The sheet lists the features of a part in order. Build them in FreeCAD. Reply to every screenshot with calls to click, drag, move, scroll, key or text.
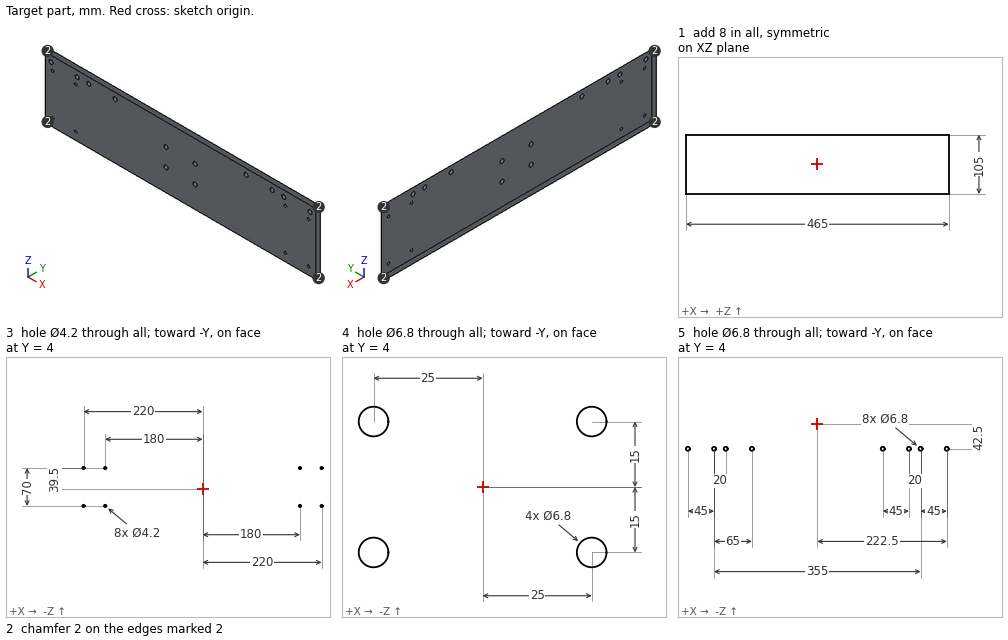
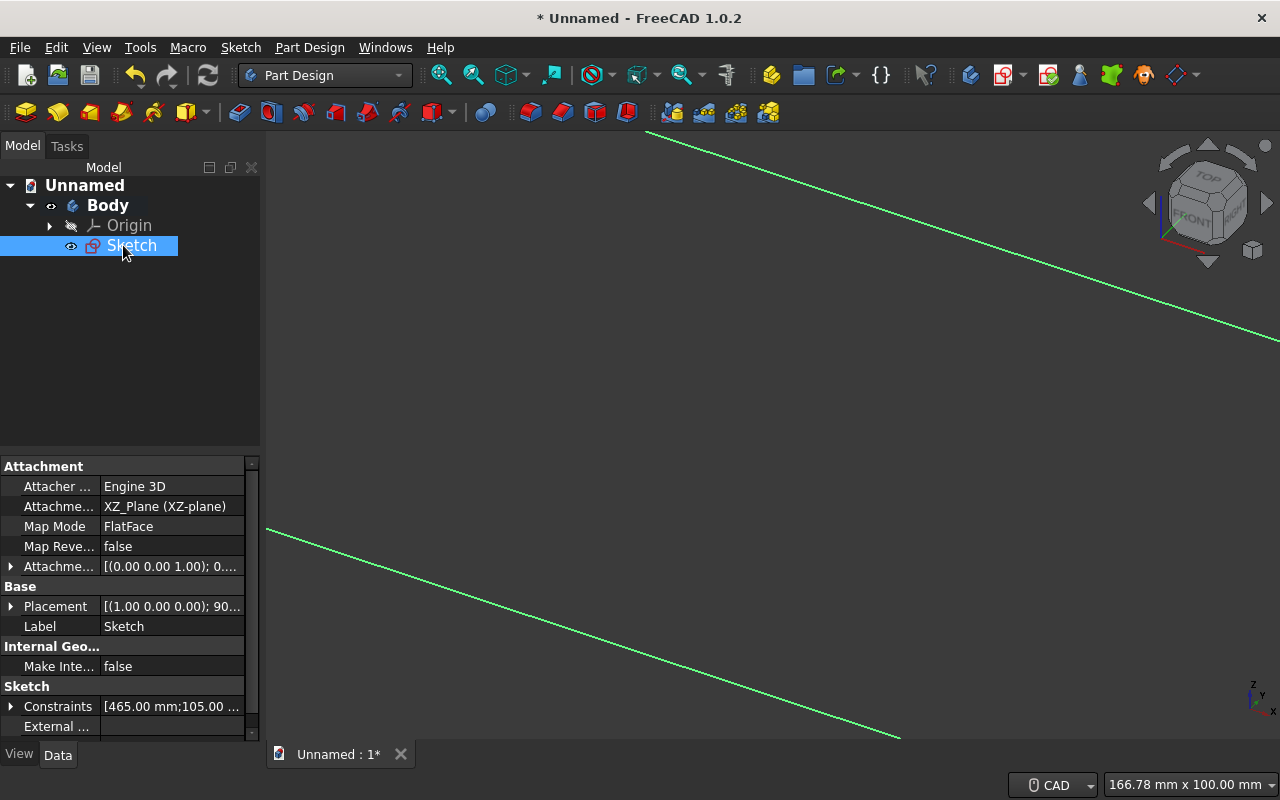
click(26, 112)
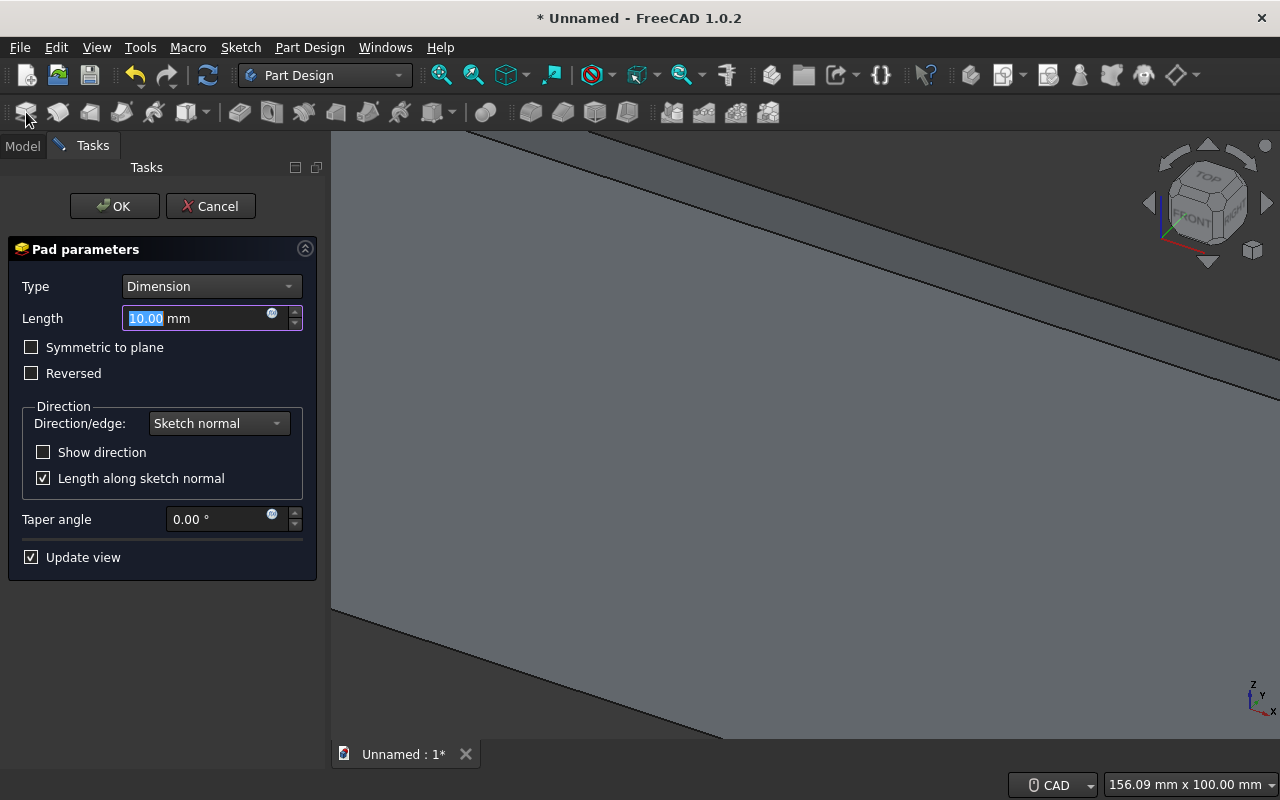
text(8)
key(Tab)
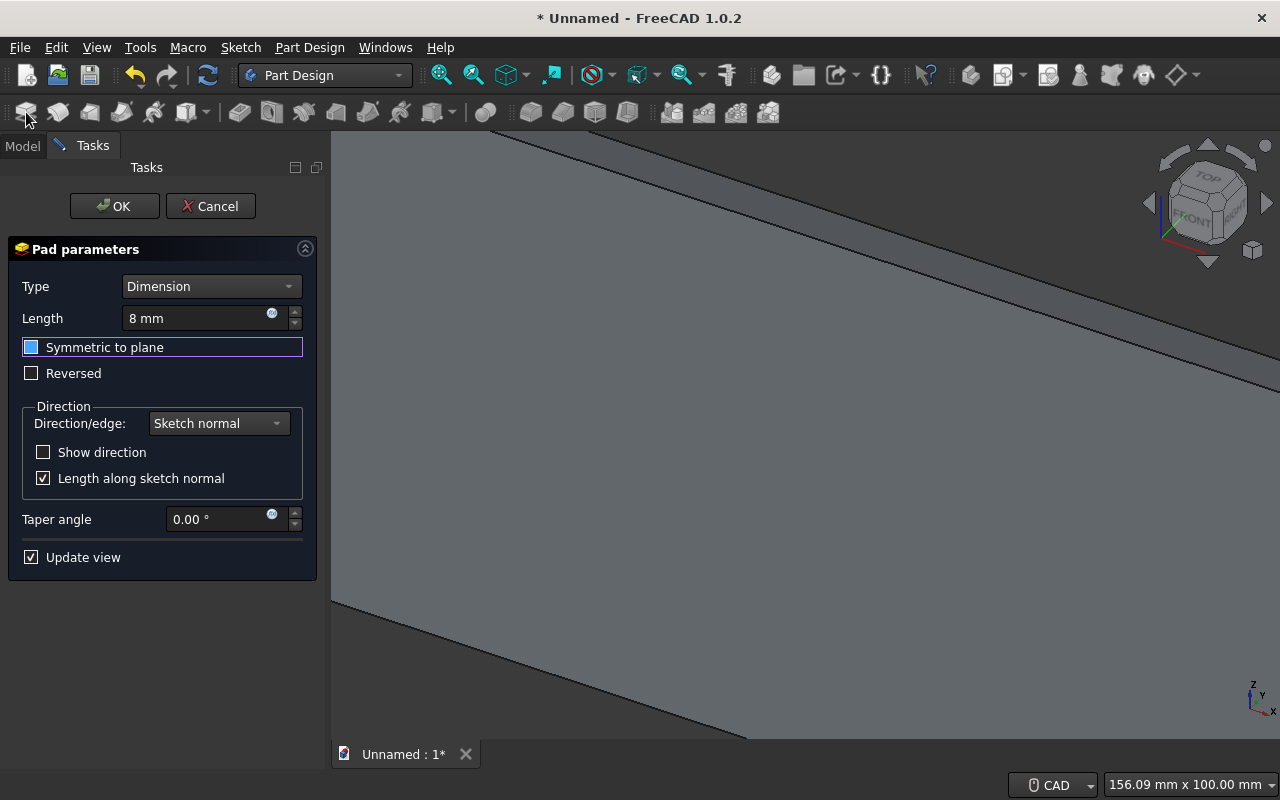
click(30, 347)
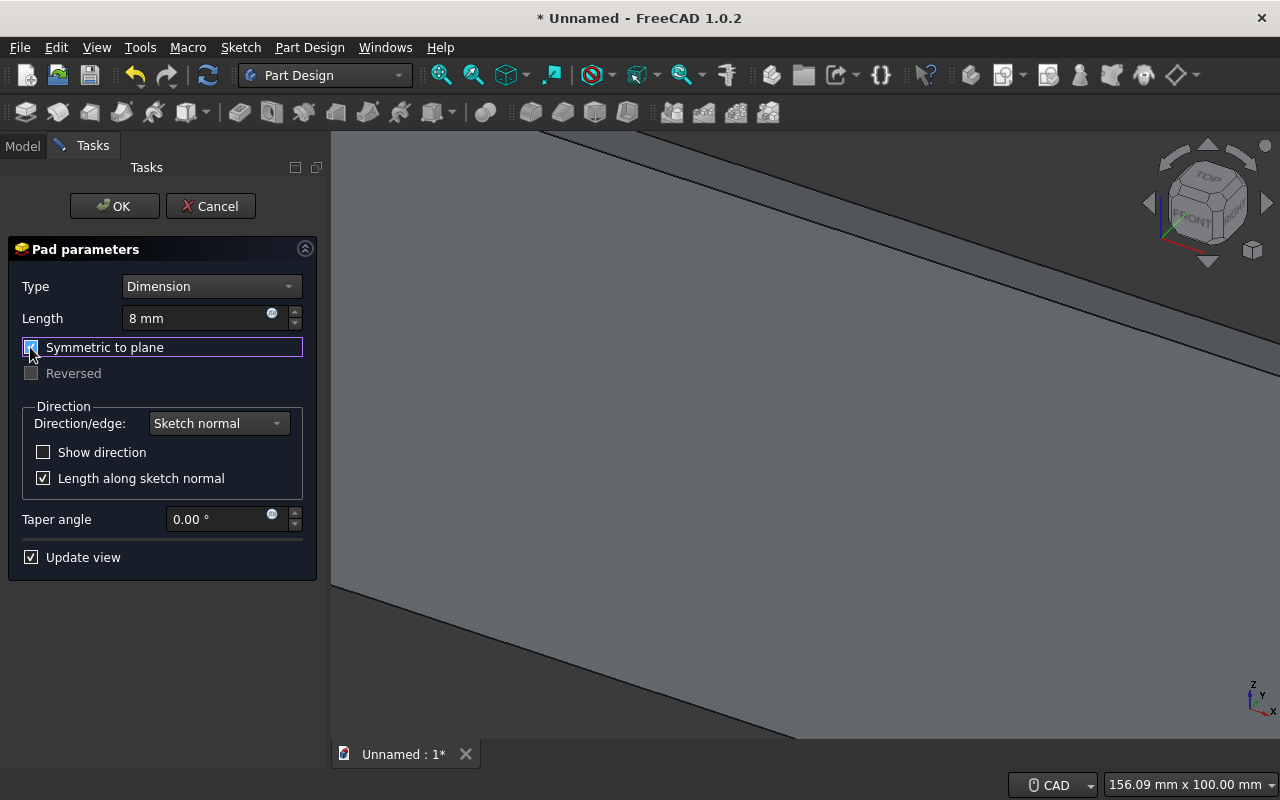
click(115, 206)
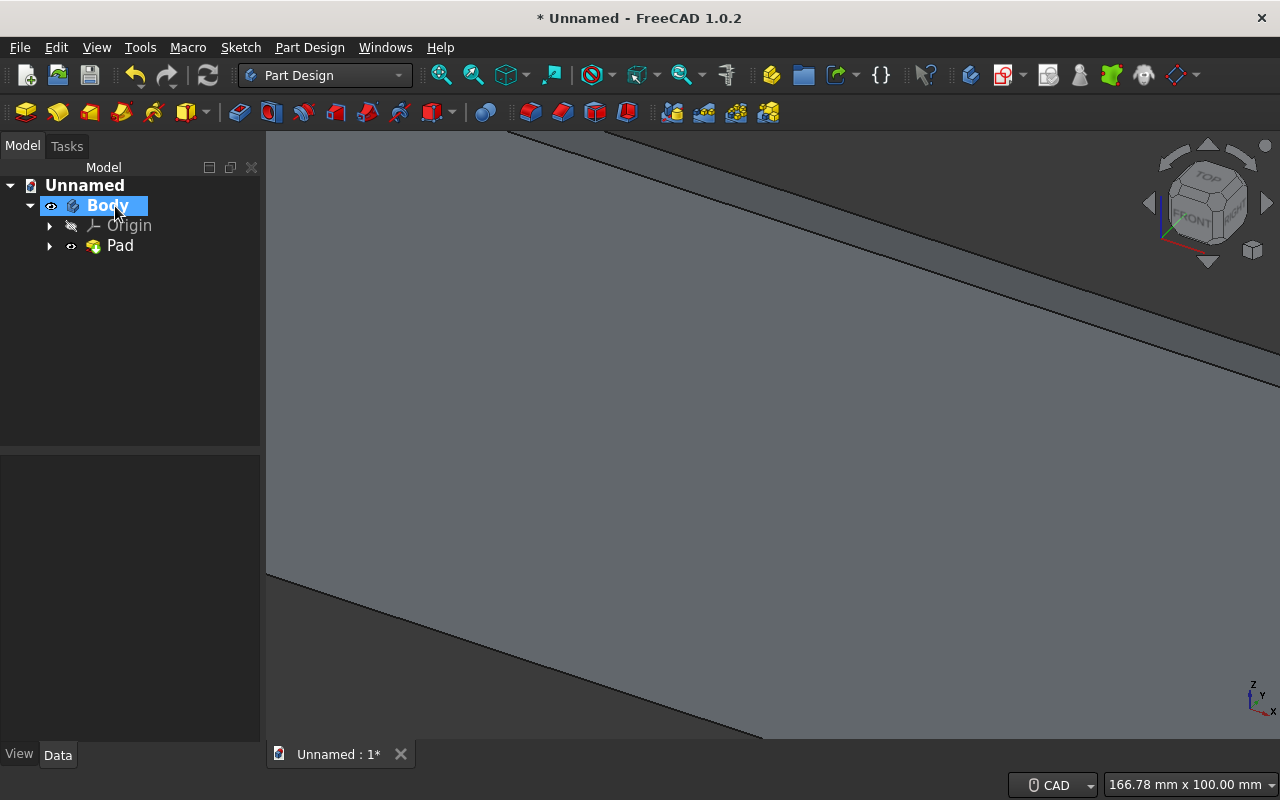
click(442, 76)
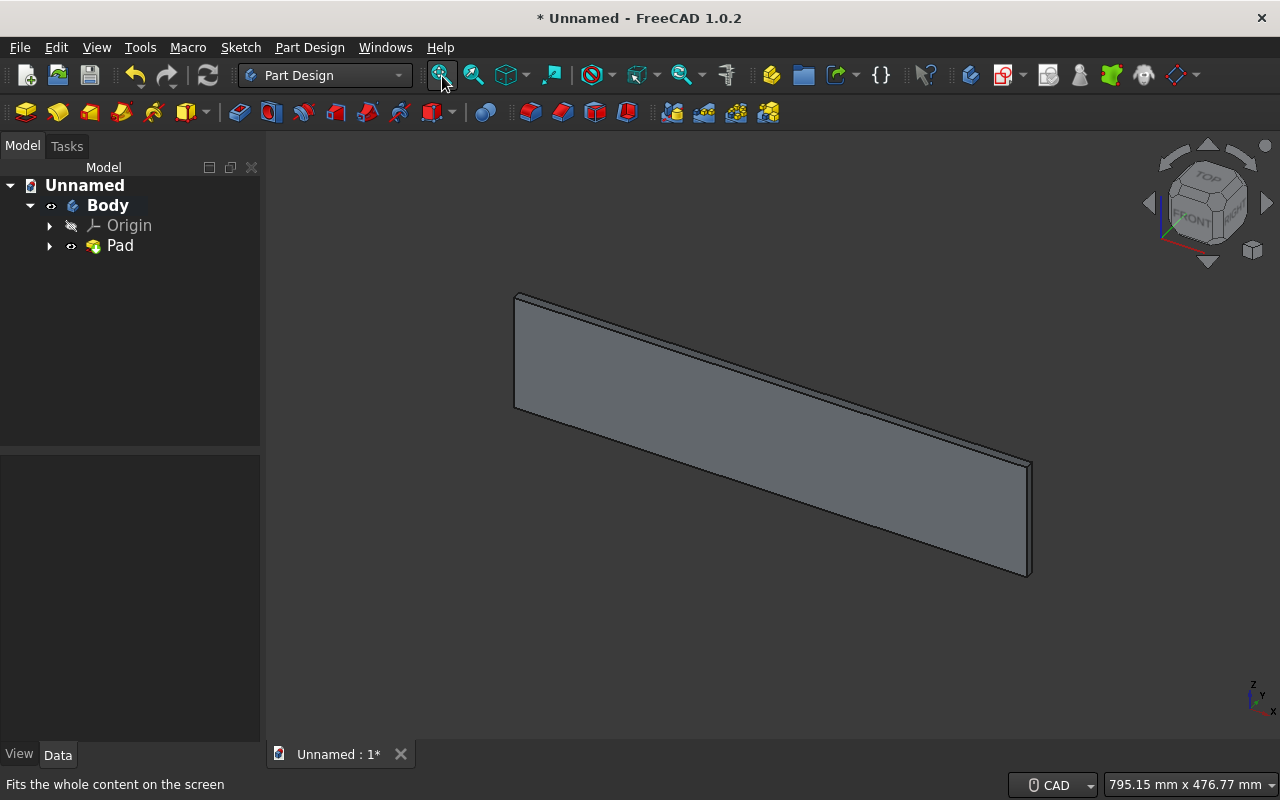
scroll(1030, 464, up, 7)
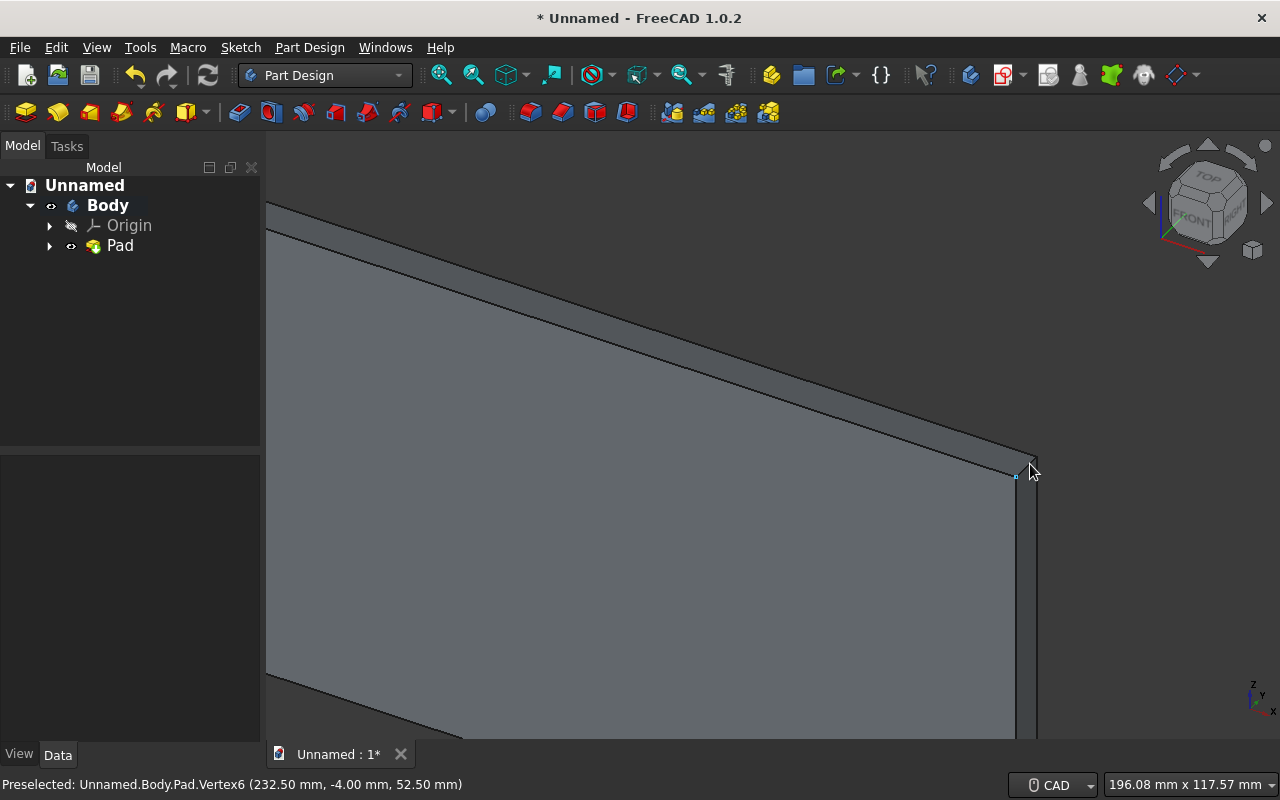
click(1027, 466)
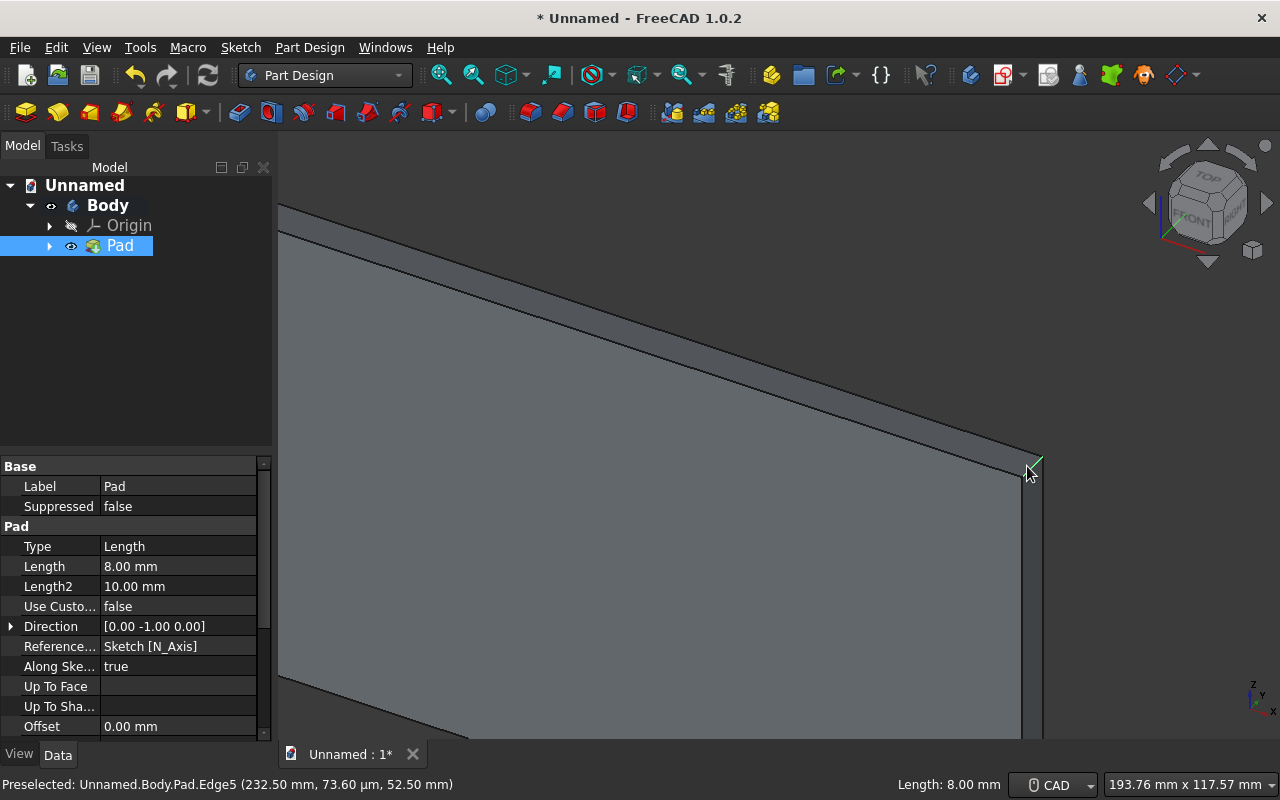
click(442, 76)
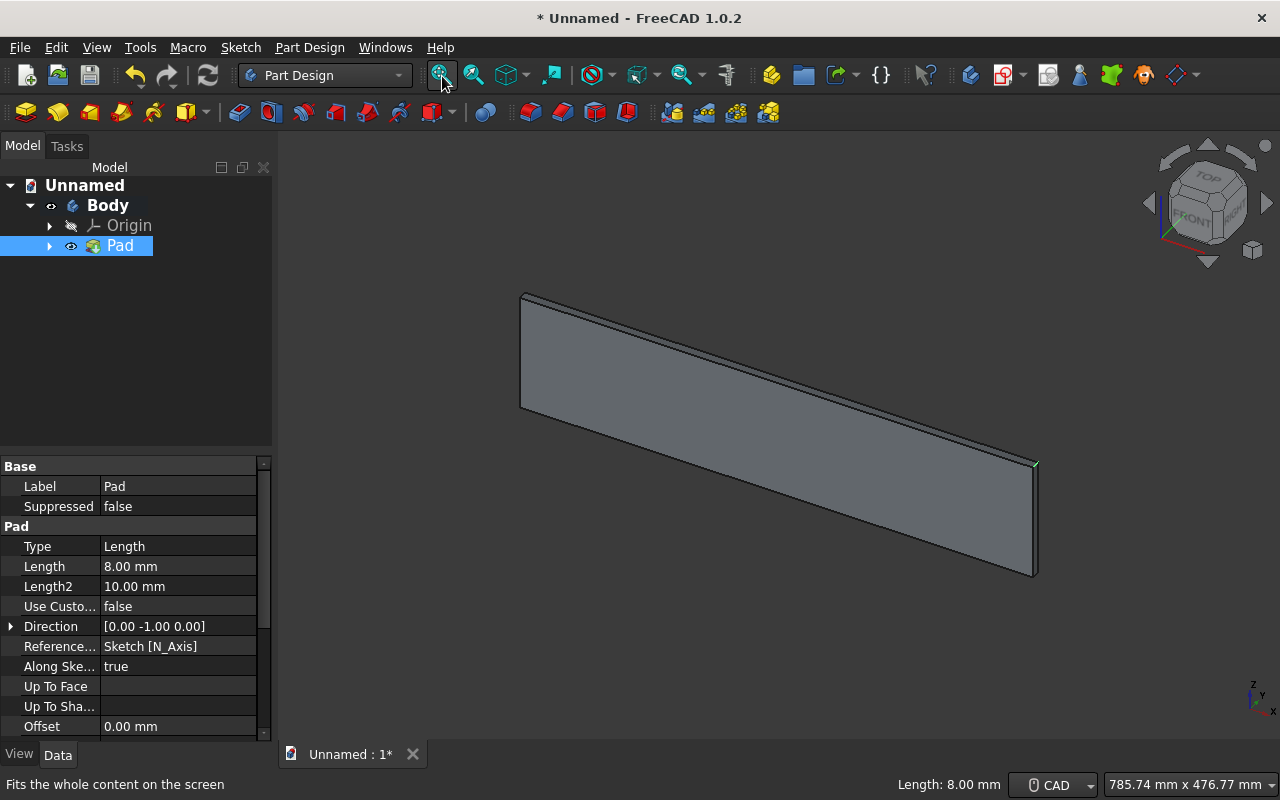
key(0)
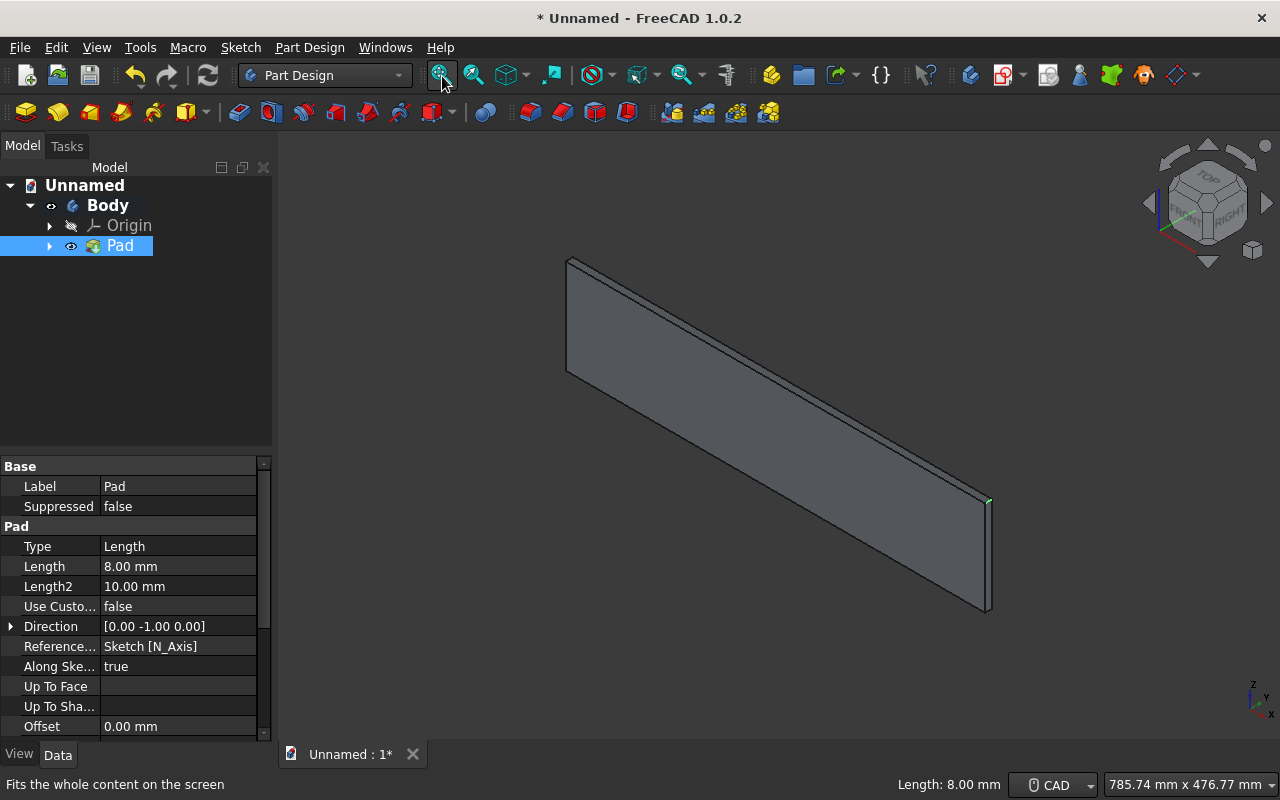
scroll(569, 258, up, 7)